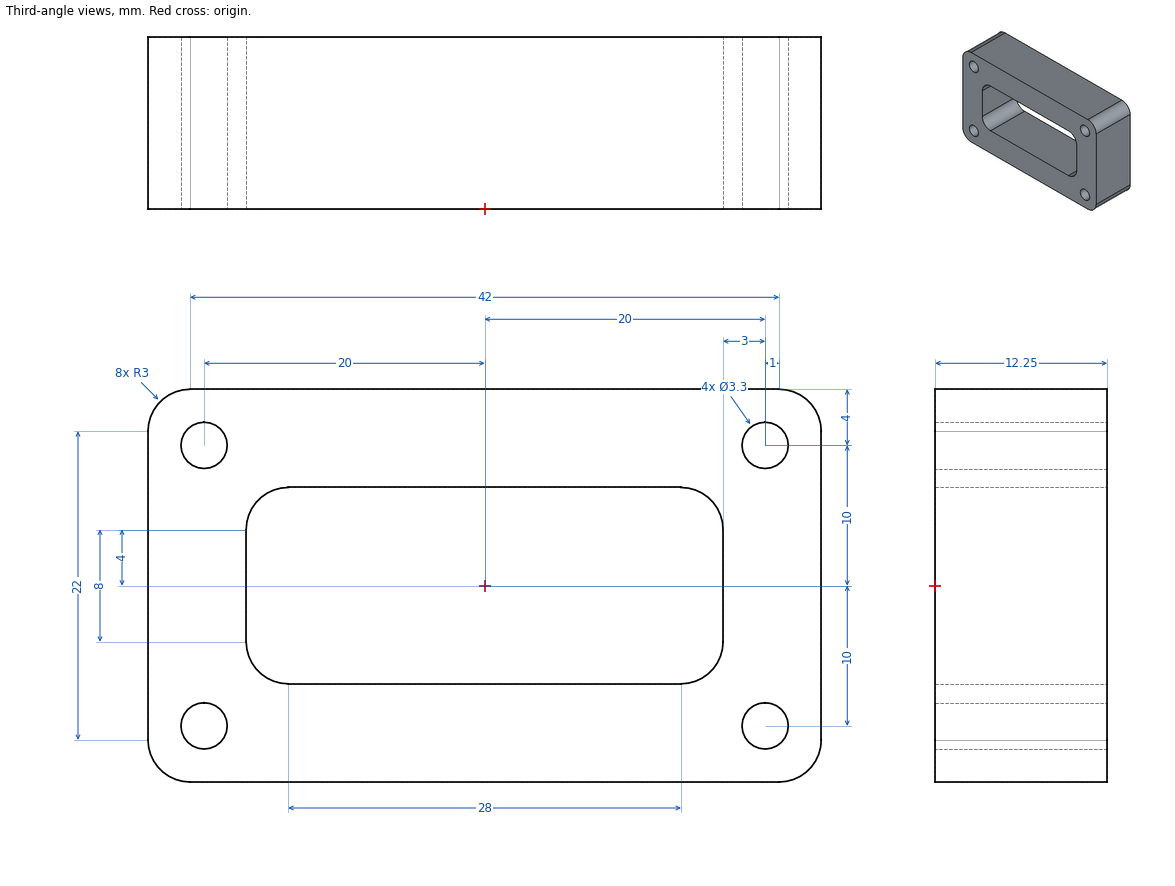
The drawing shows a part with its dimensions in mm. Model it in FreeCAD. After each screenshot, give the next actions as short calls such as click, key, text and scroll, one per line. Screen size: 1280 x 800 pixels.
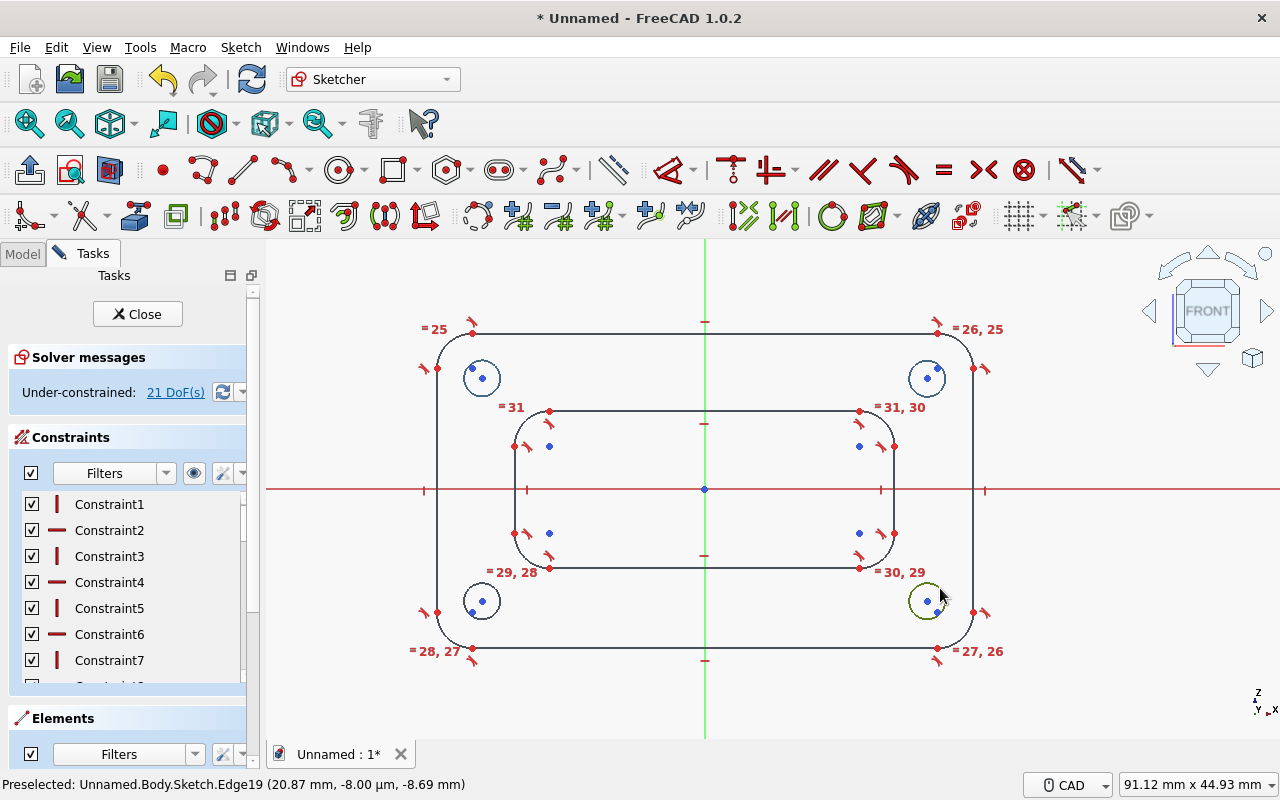
click(495, 588)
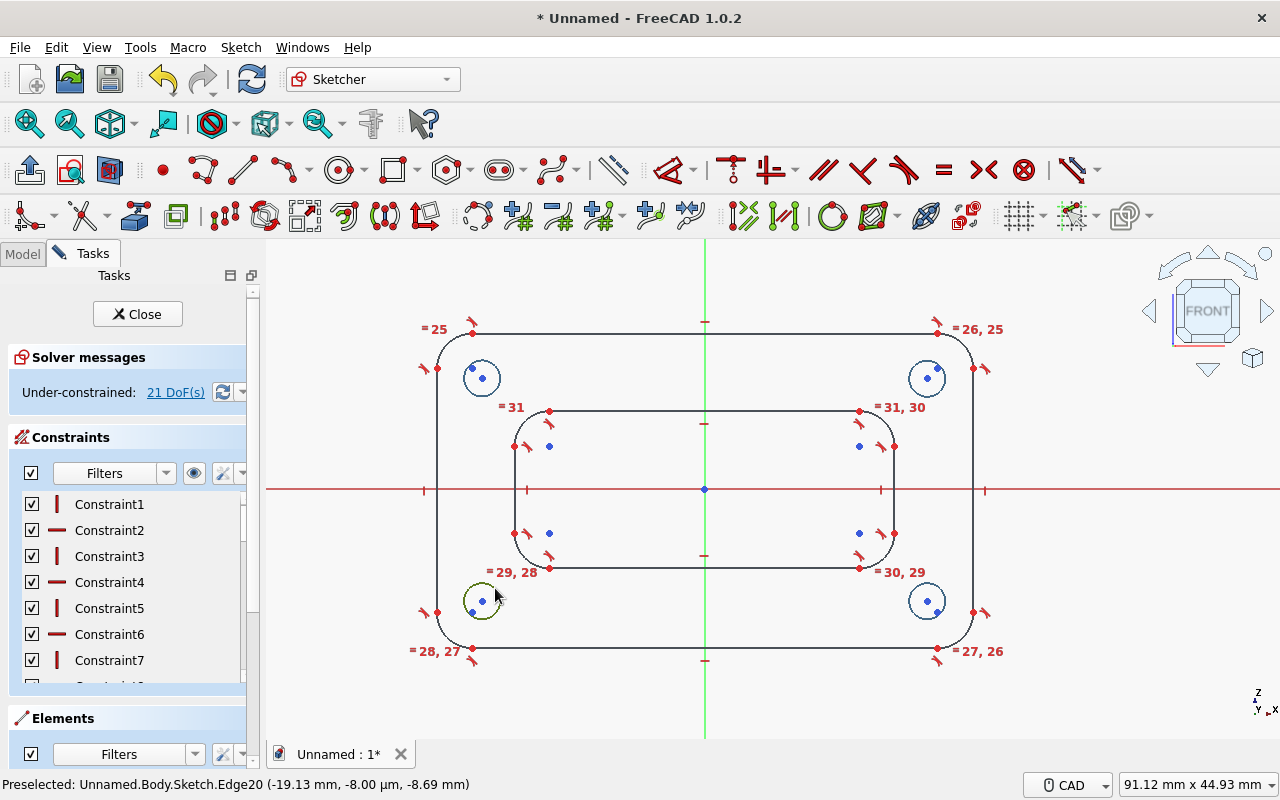
click(944, 170)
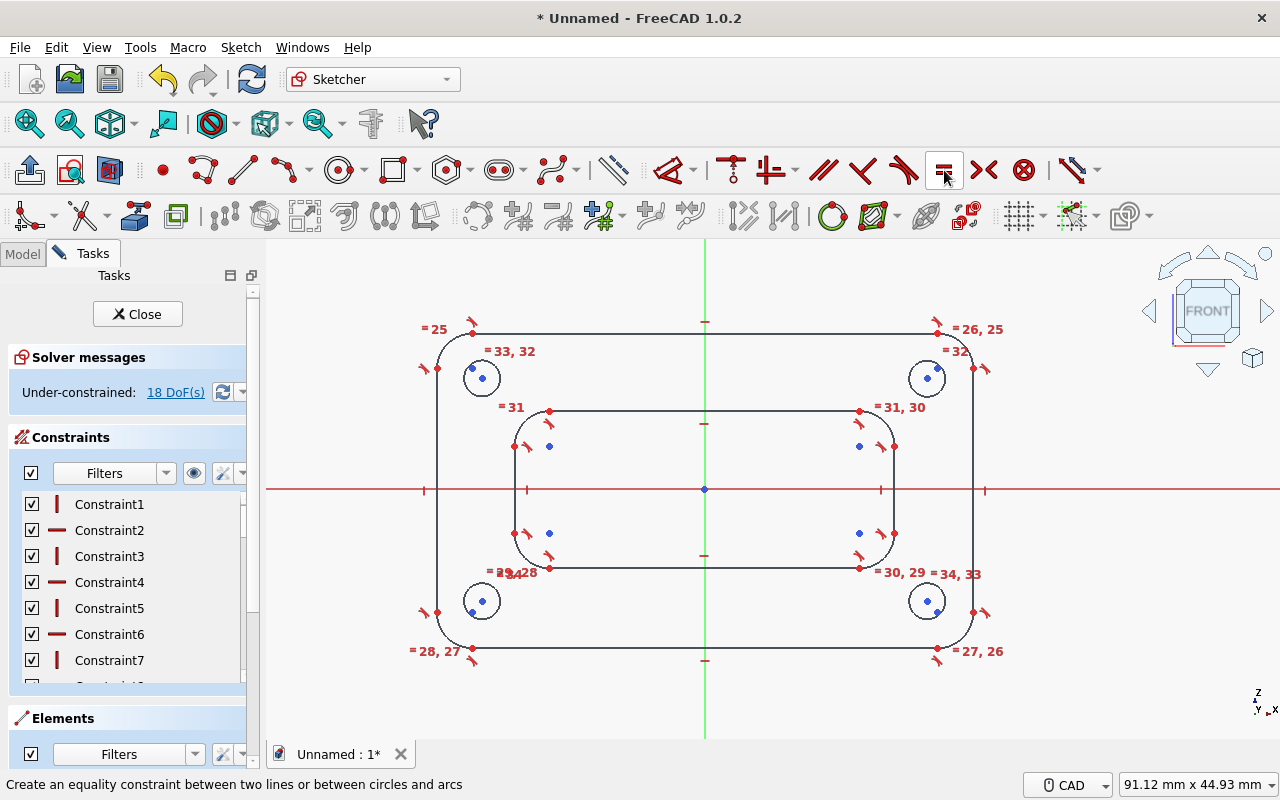
click(668, 170)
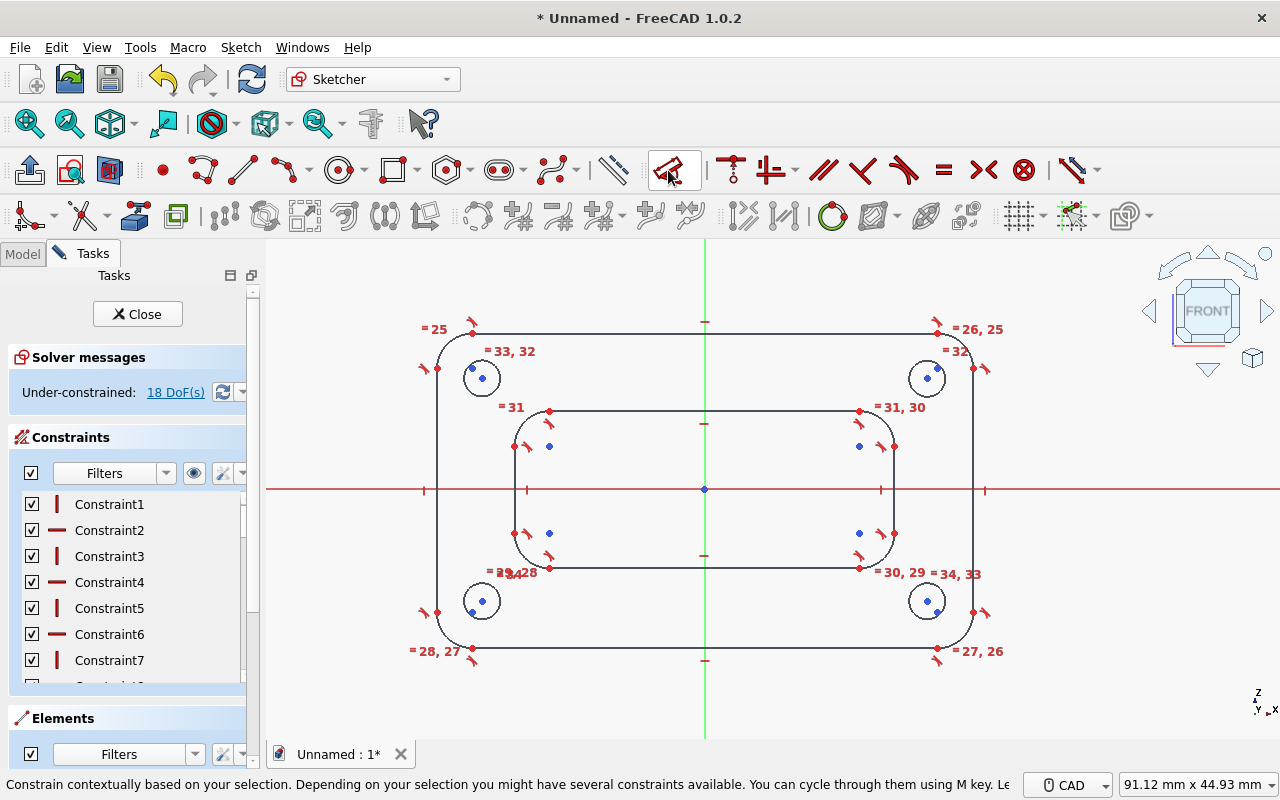
click(456, 338)
click(441, 310)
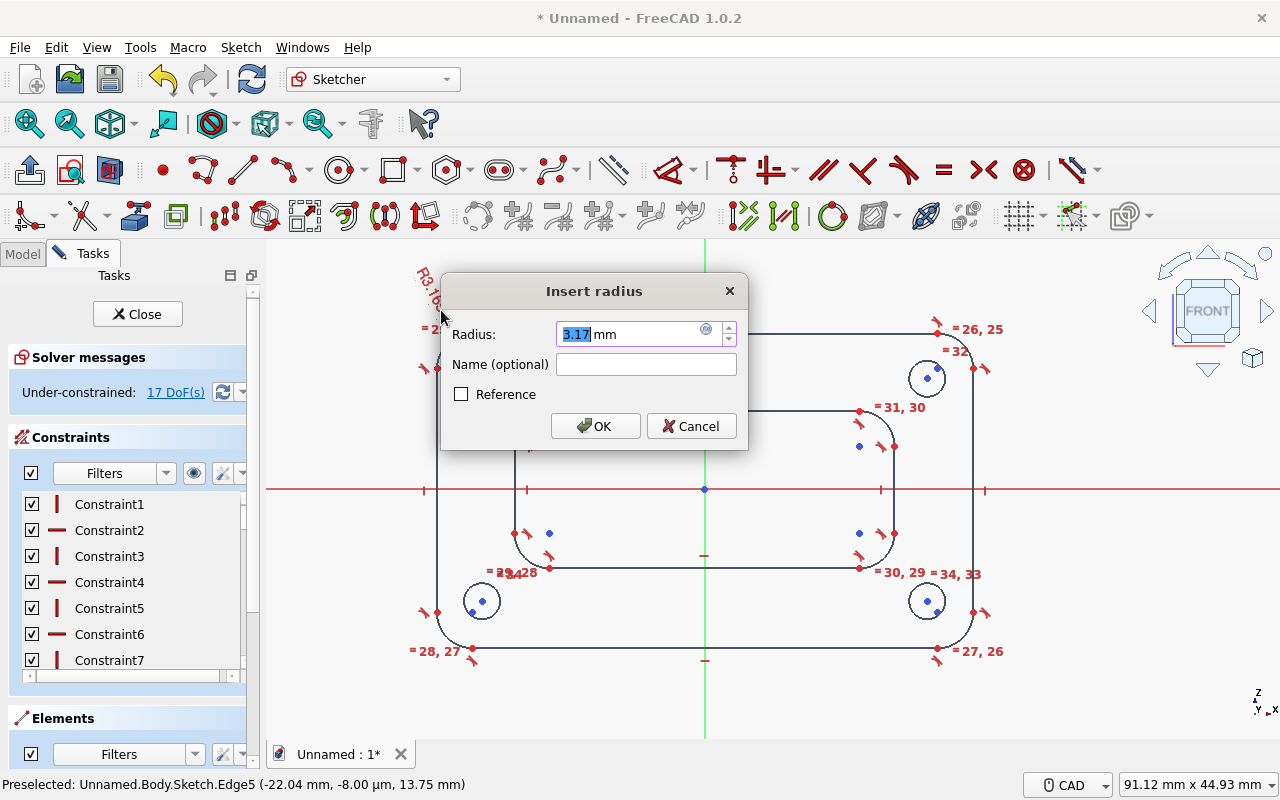
text(3)
key(Return)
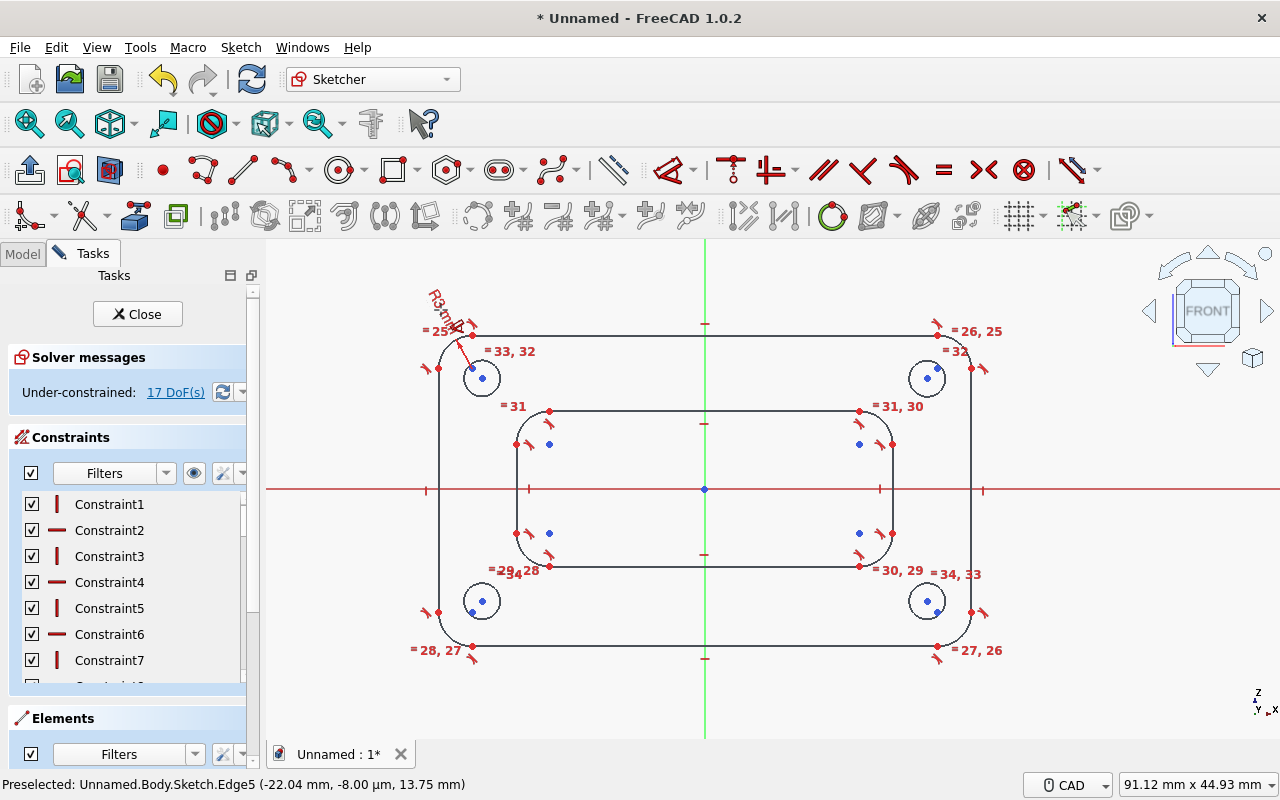
click(914, 366)
click(879, 365)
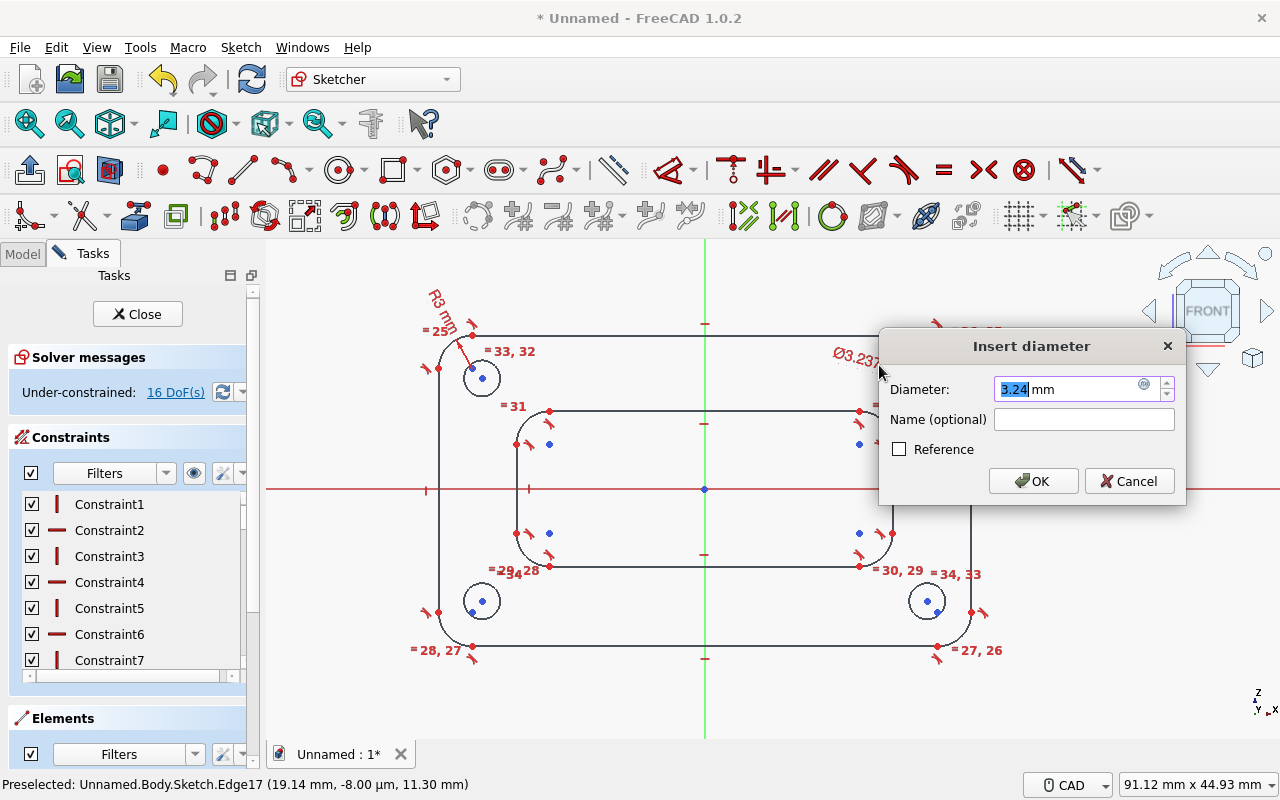
text(3.3)
key(Return)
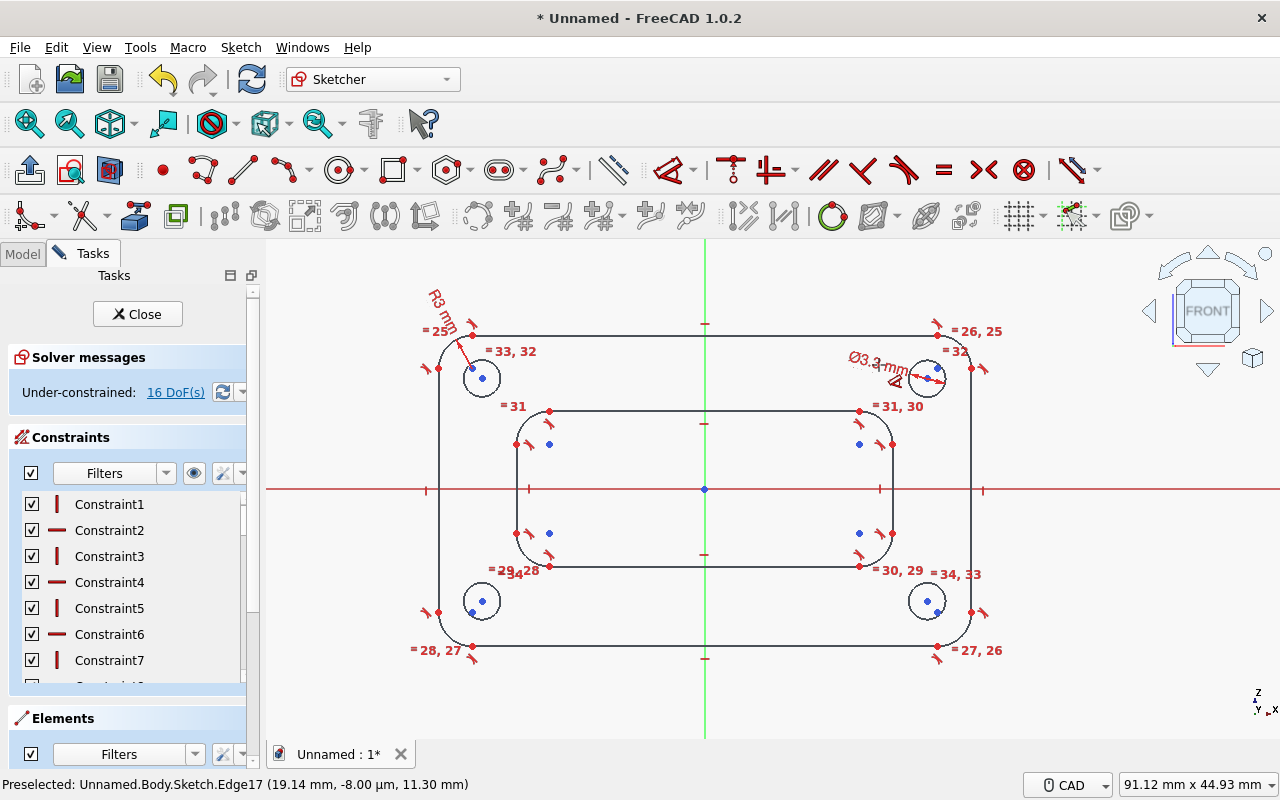
click(517, 471)
click(483, 469)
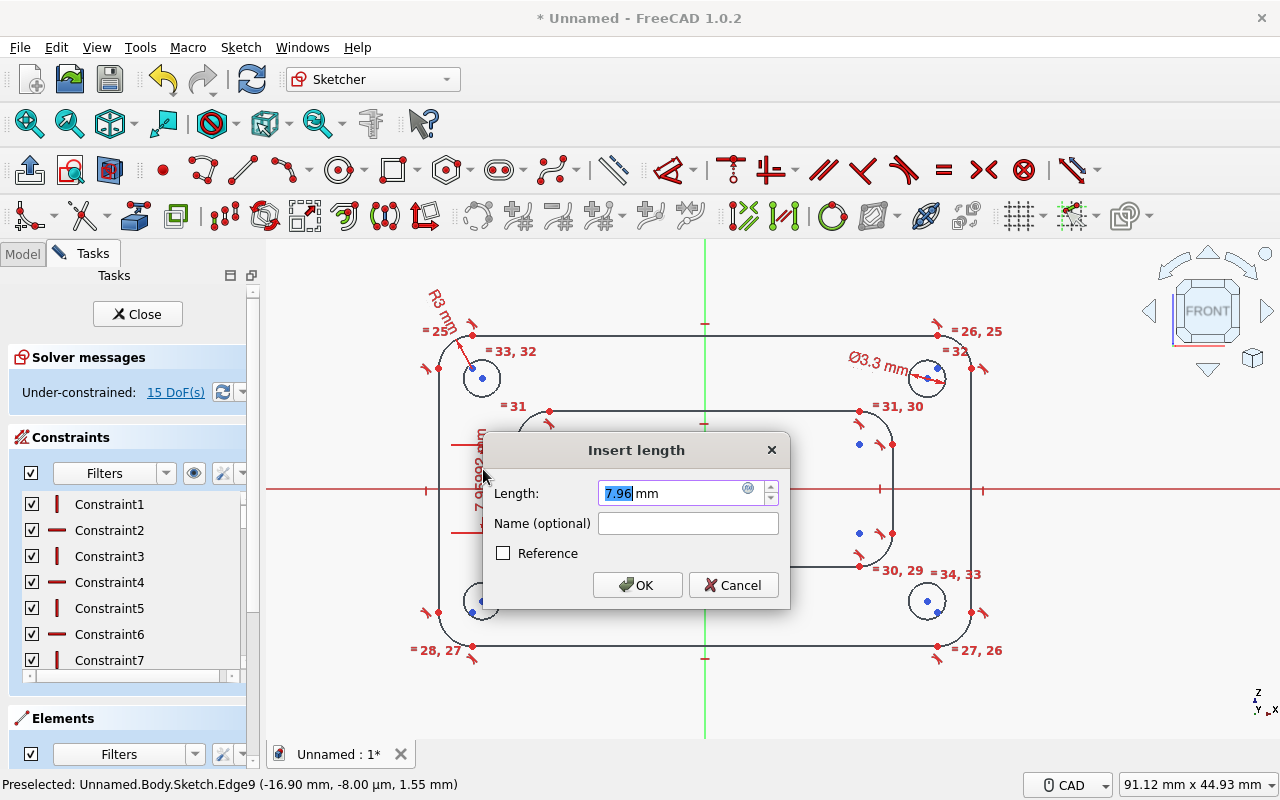
text(8)
key(Return)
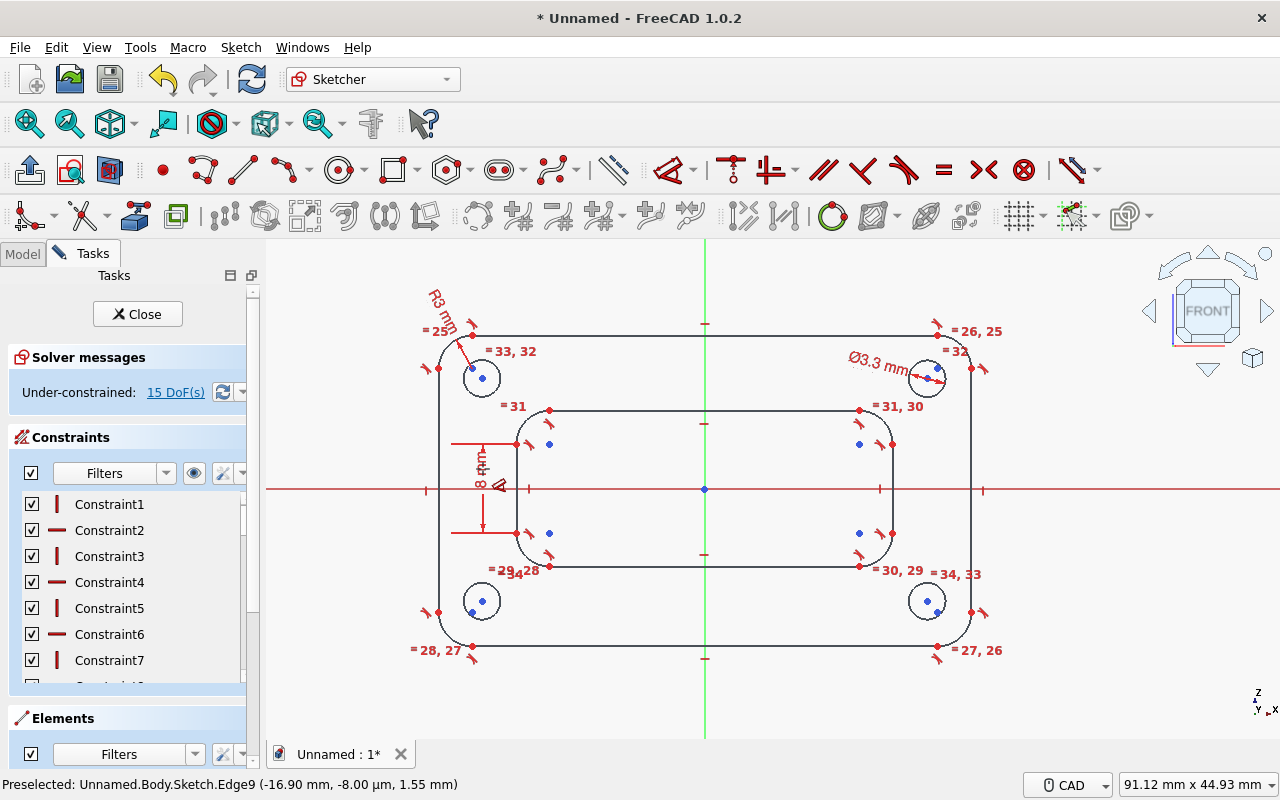
click(439, 540)
click(405, 435)